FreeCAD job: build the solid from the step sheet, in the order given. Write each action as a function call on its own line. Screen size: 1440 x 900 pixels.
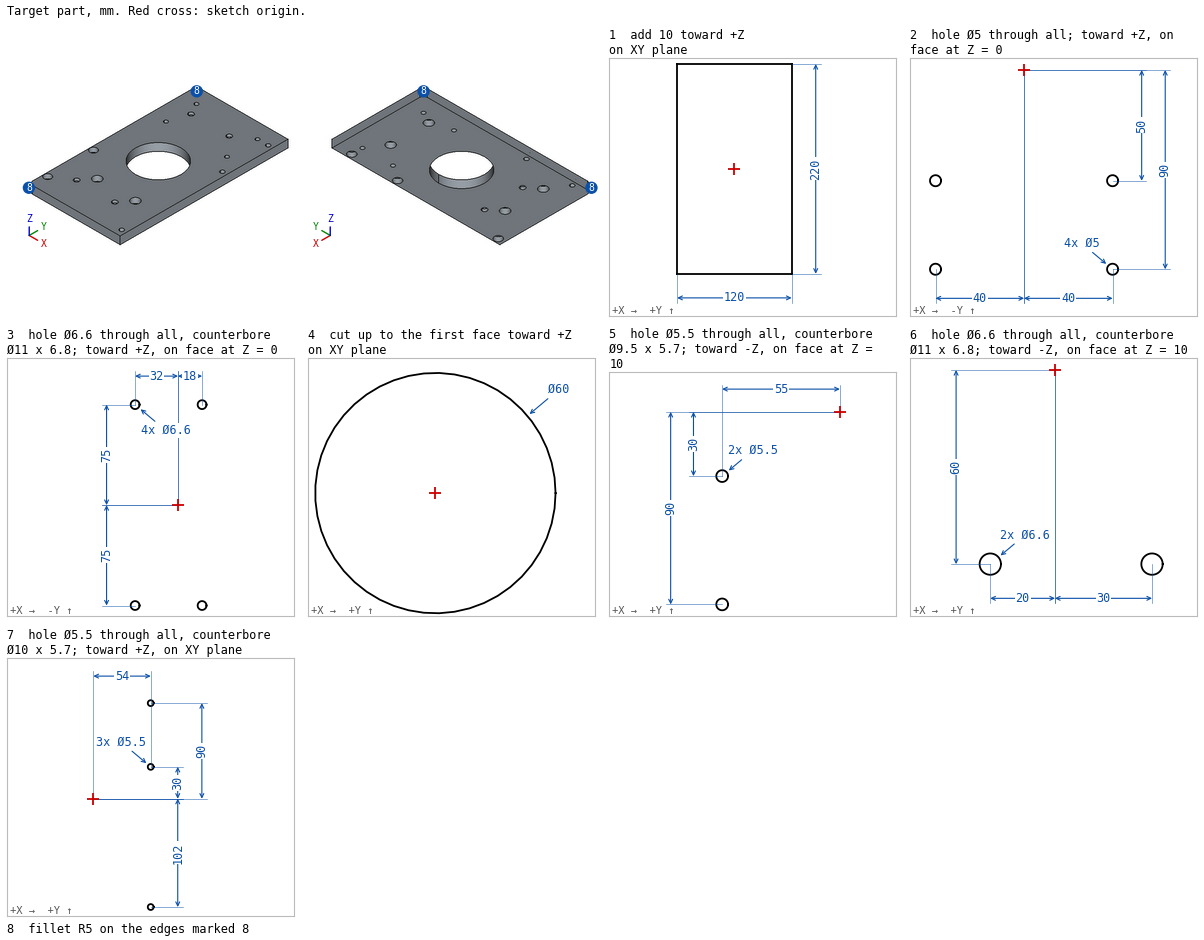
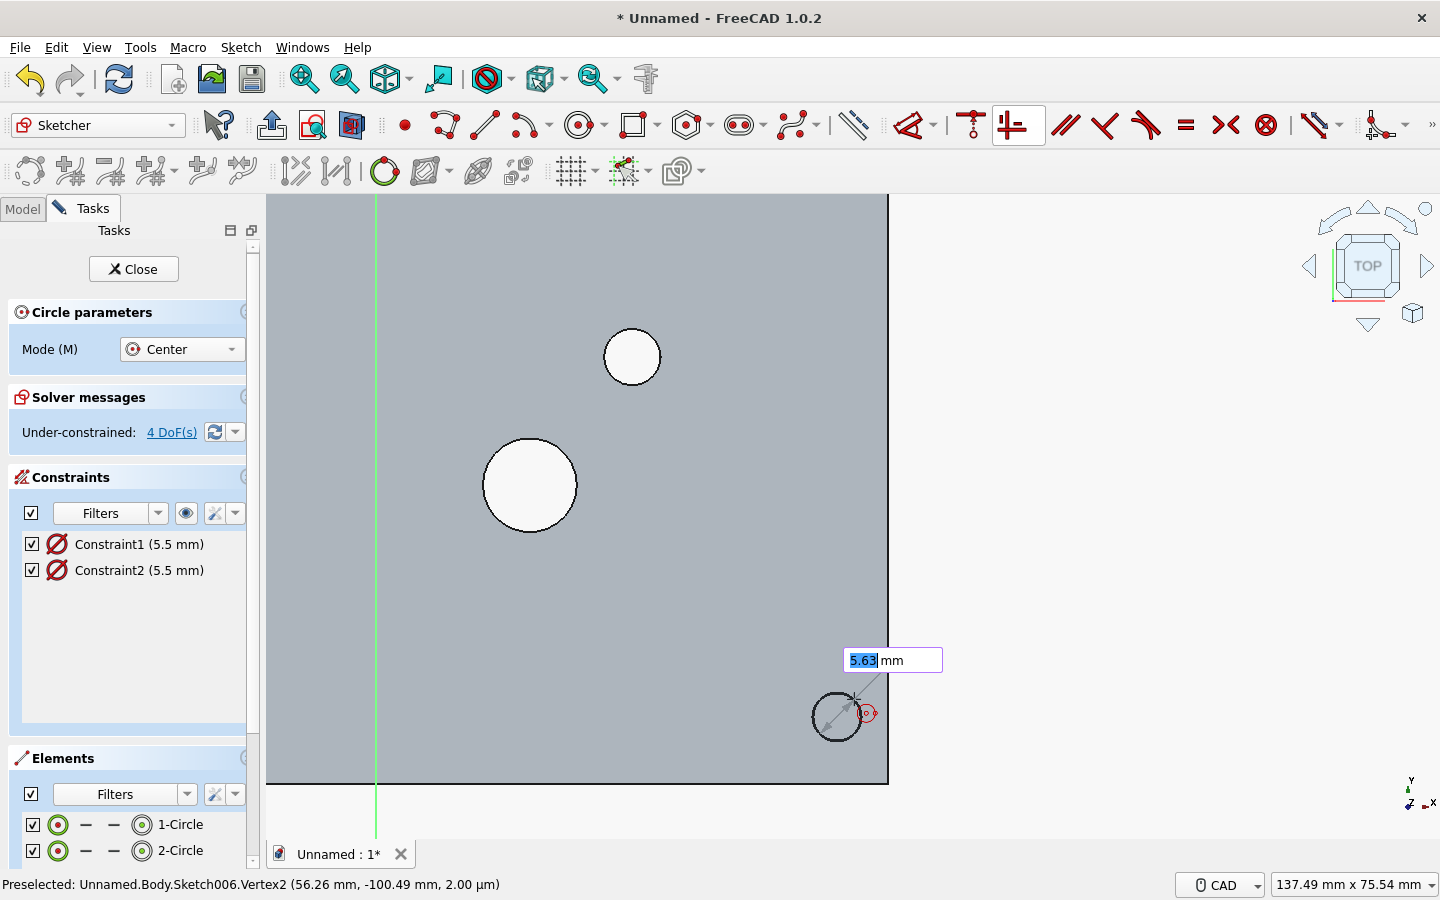
text(5.5)
key(Return)
key(Escape)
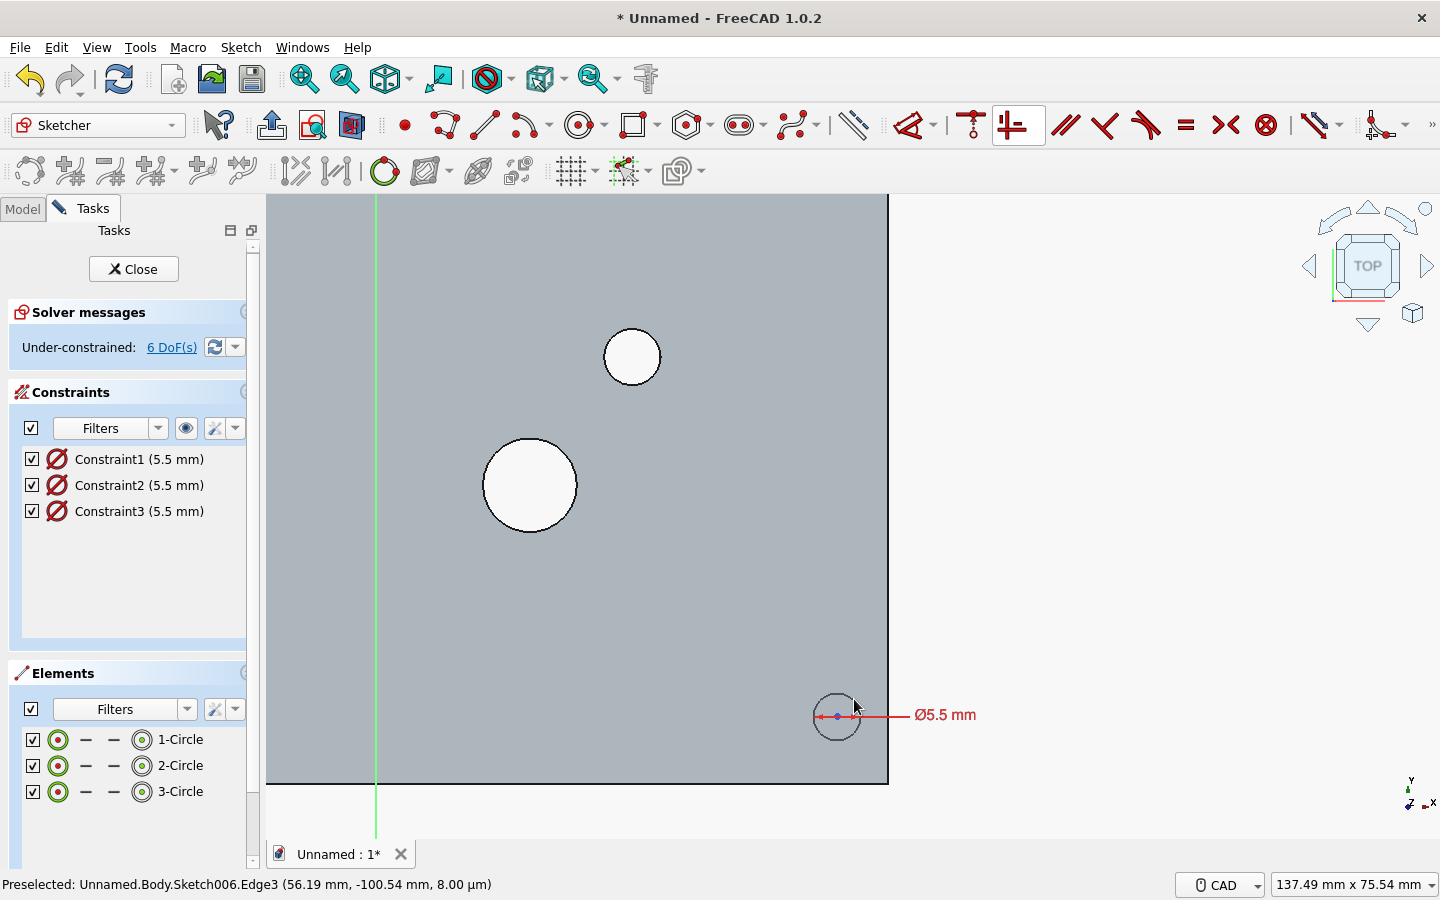
scroll(839, 720, down, 7)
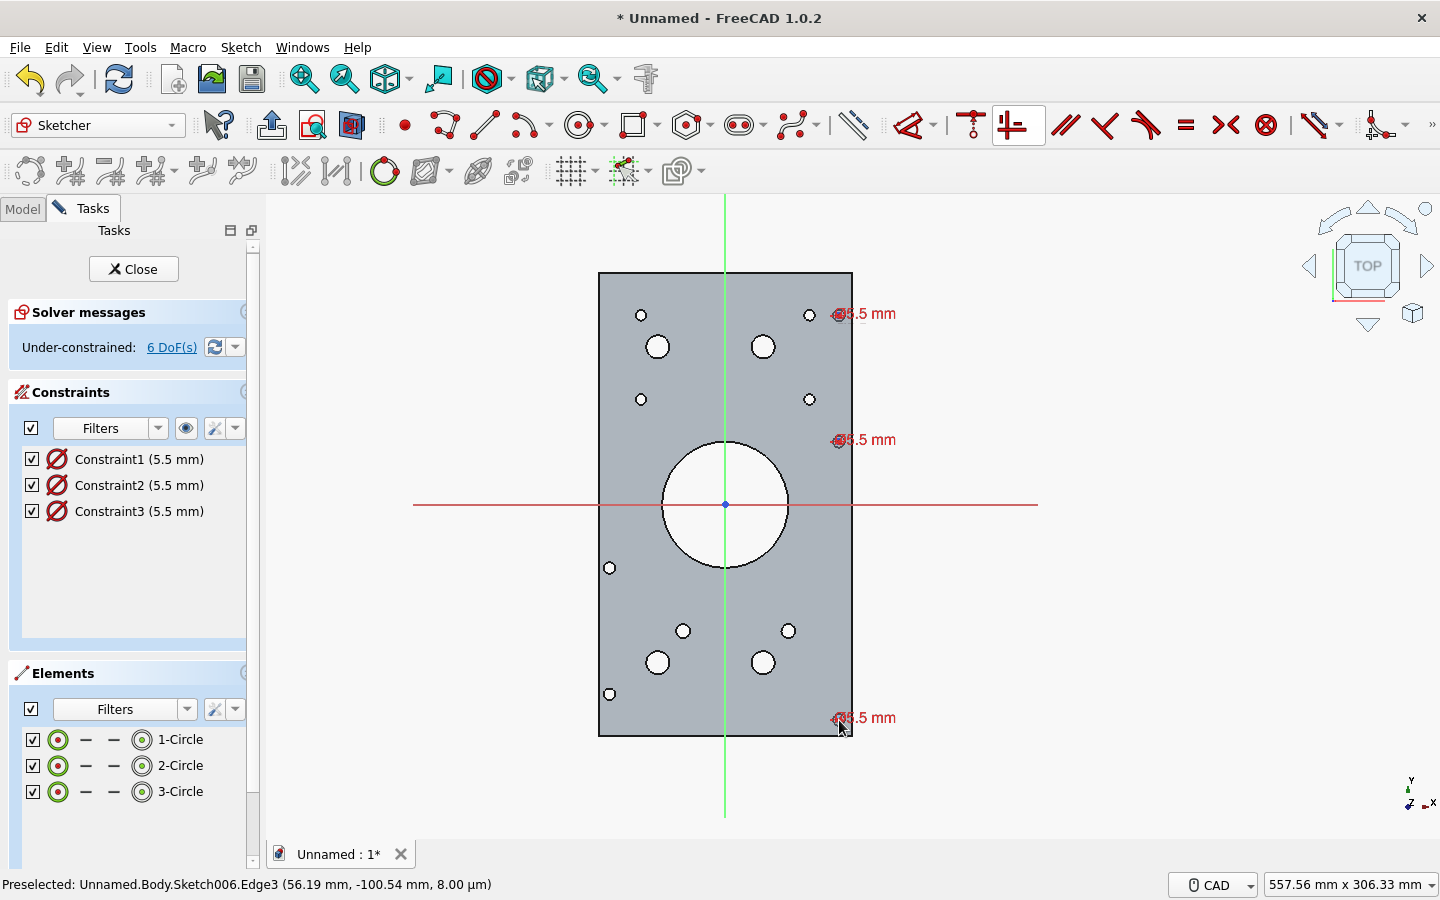
click(839, 442)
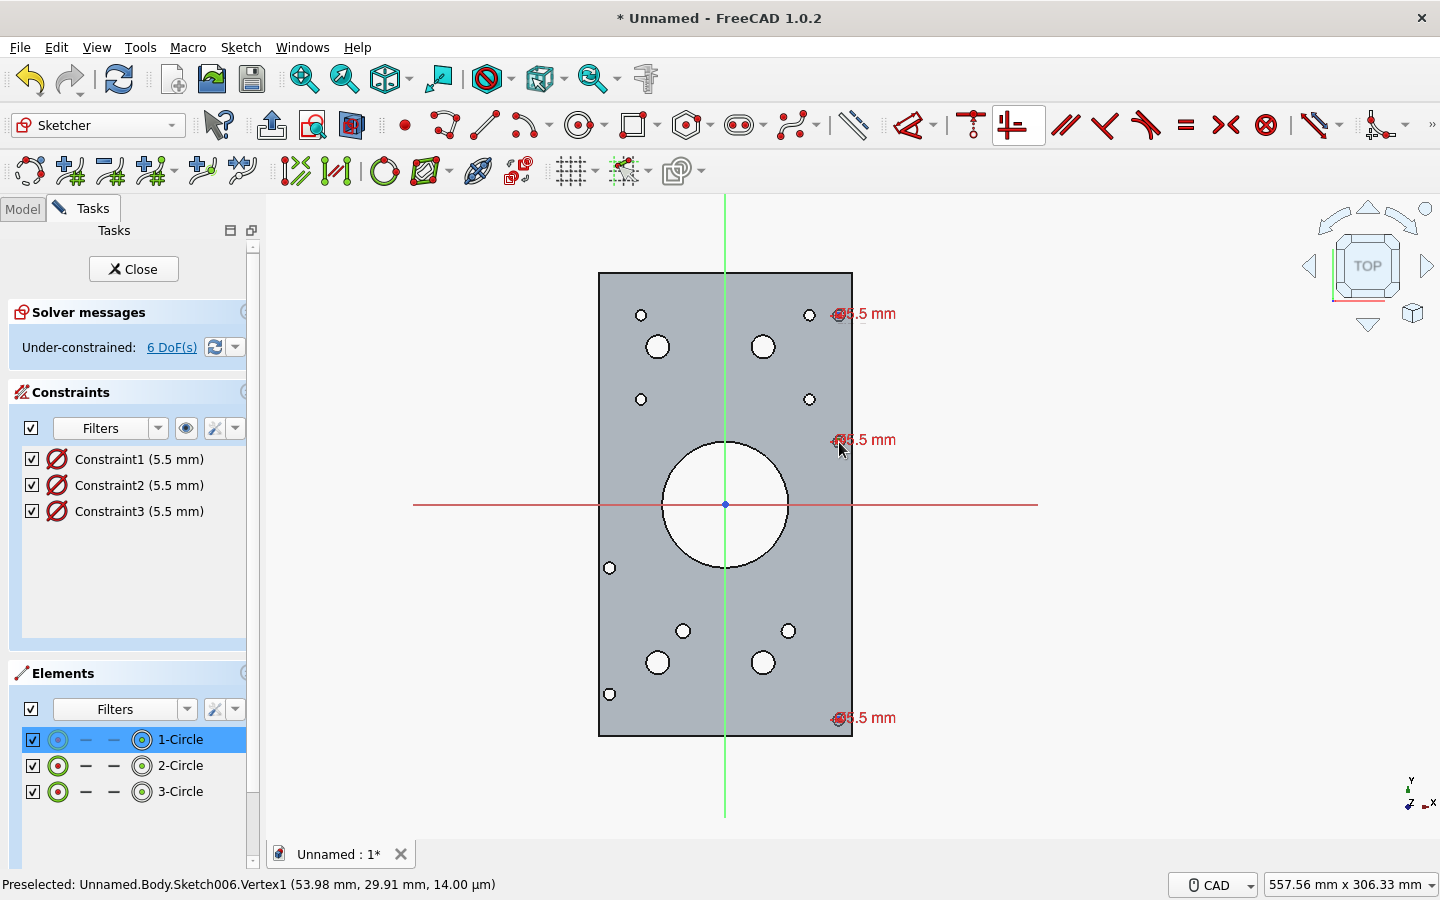
click(839, 316)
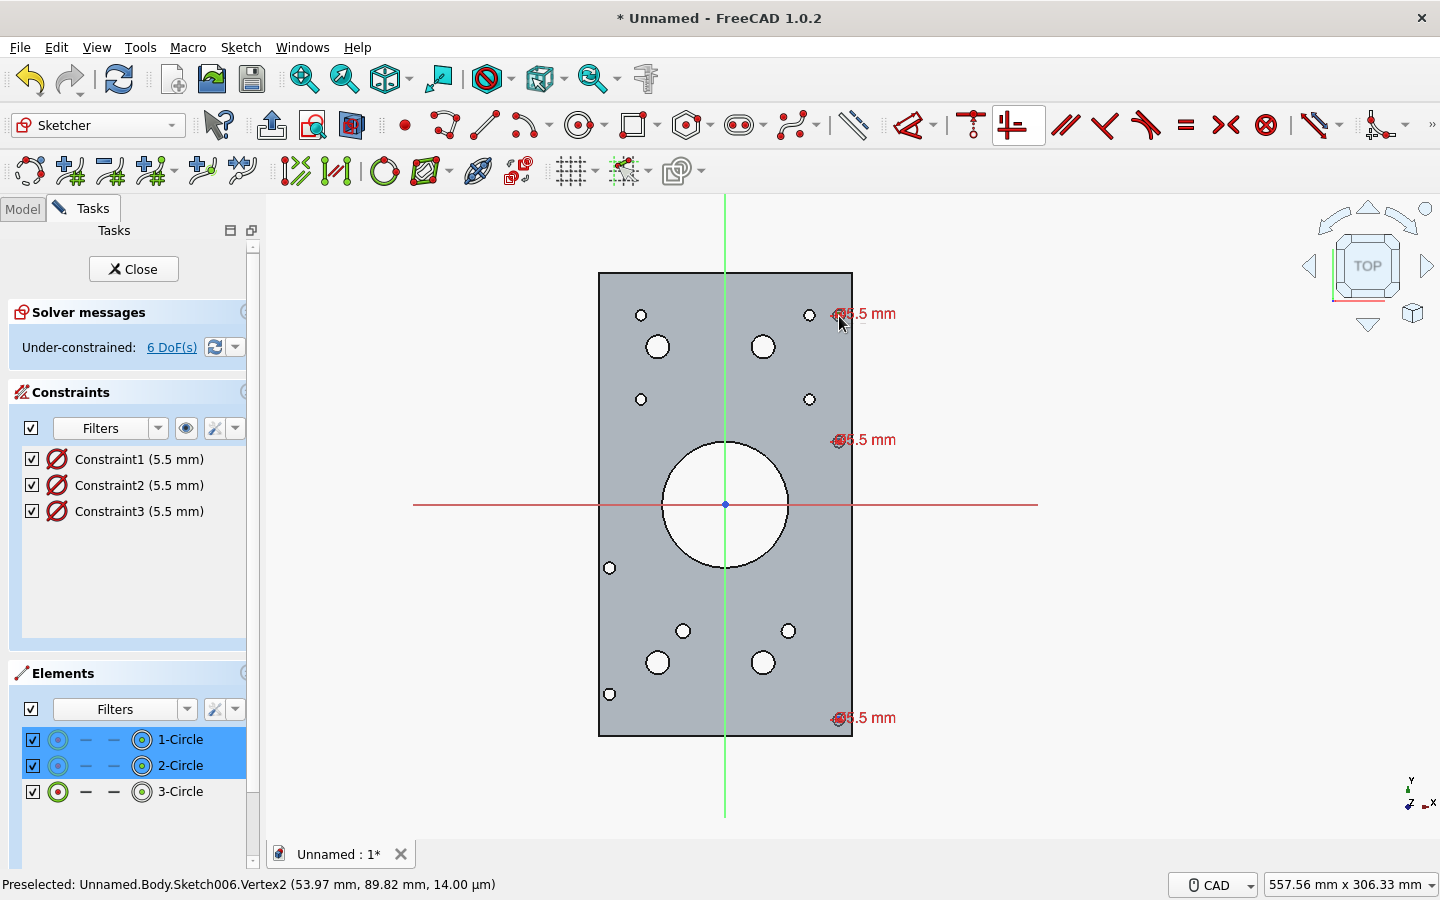
key(v)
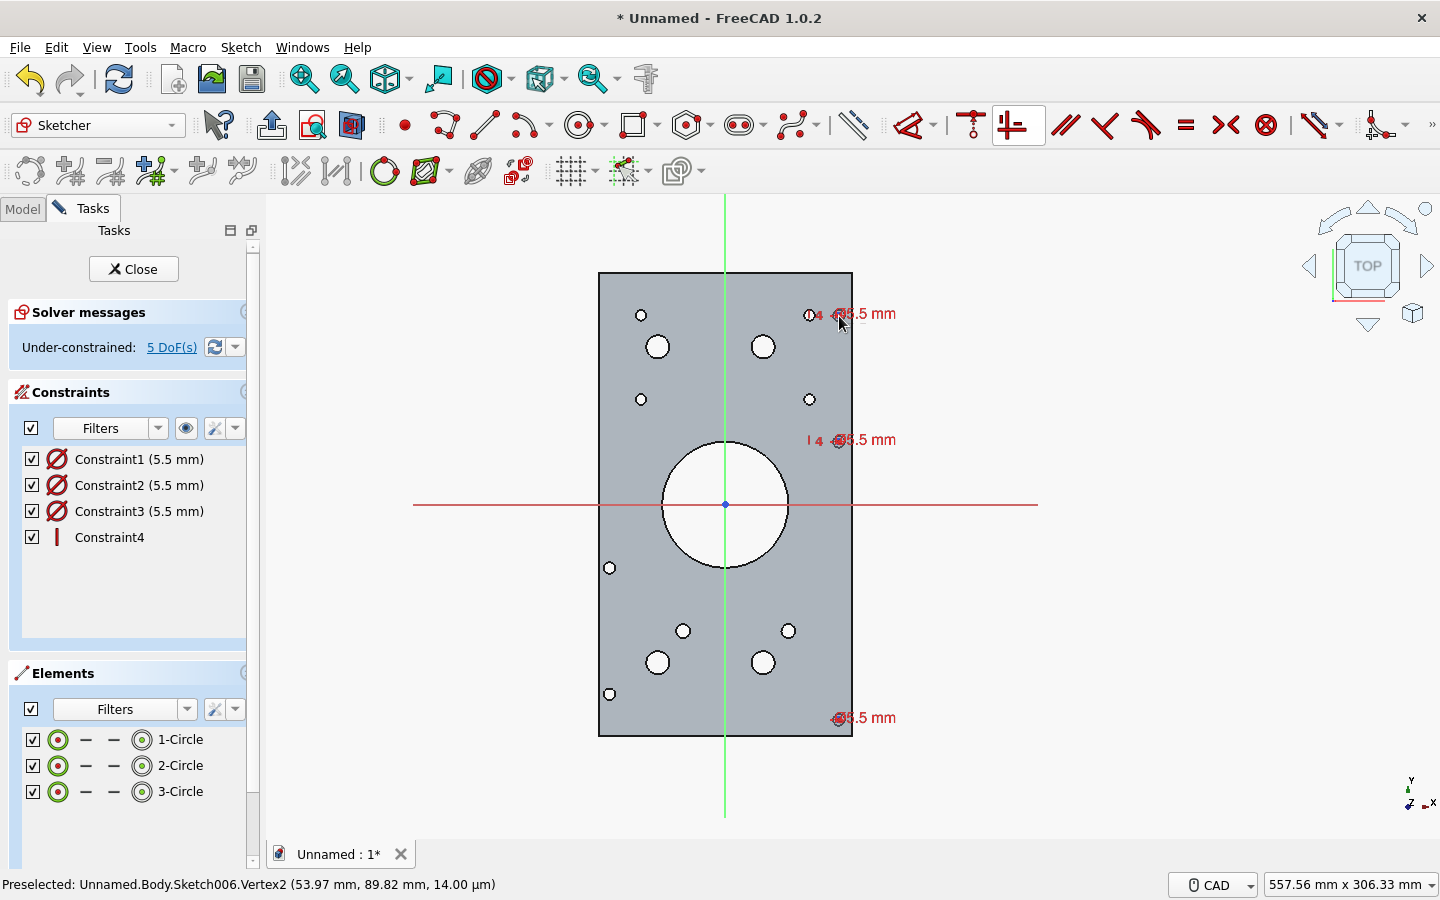
click(839, 442)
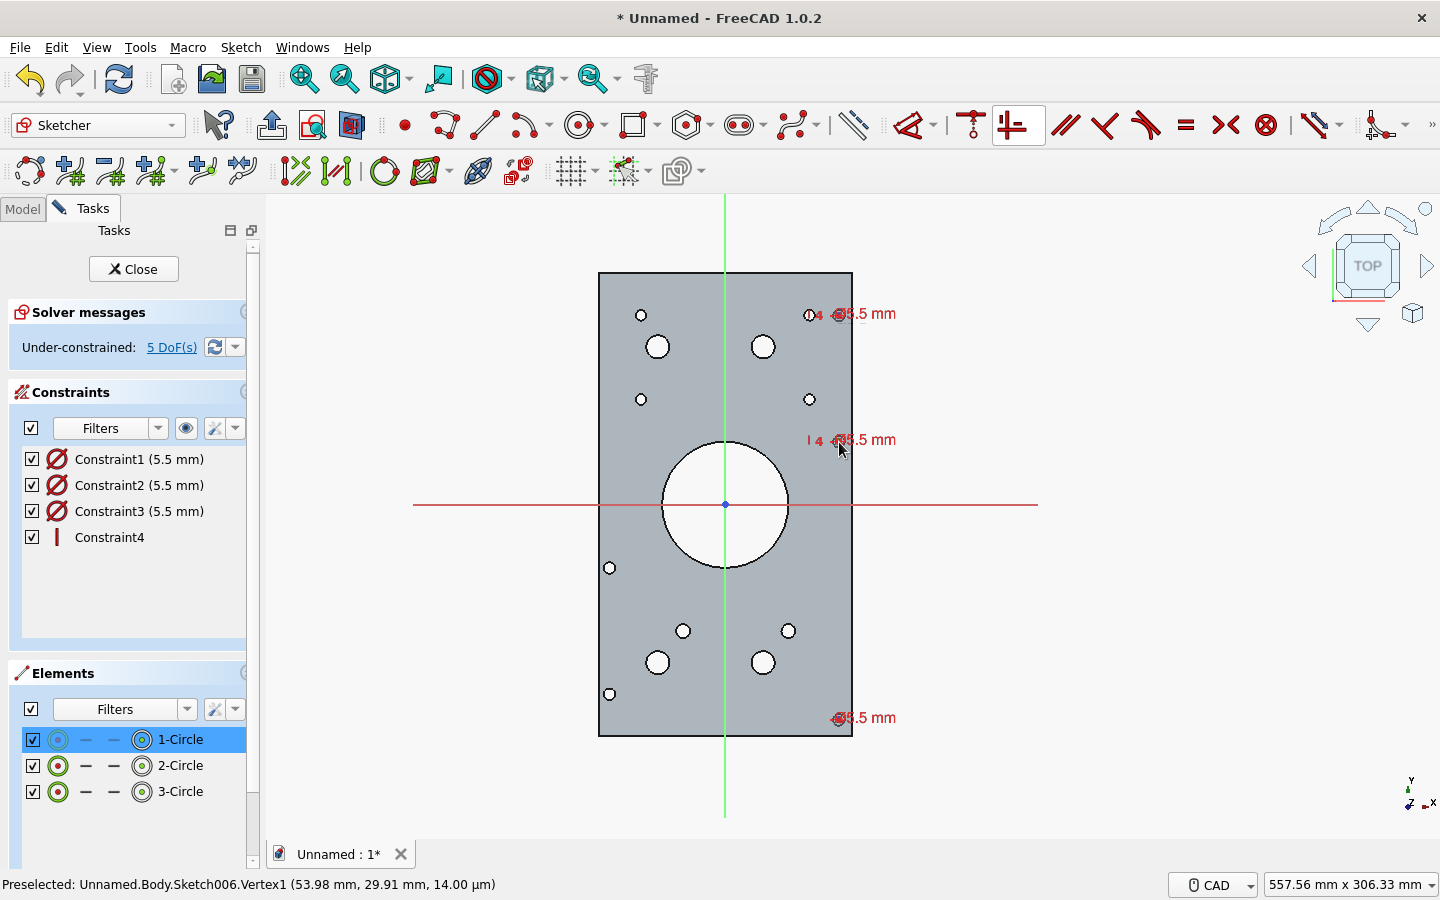
click(839, 720)